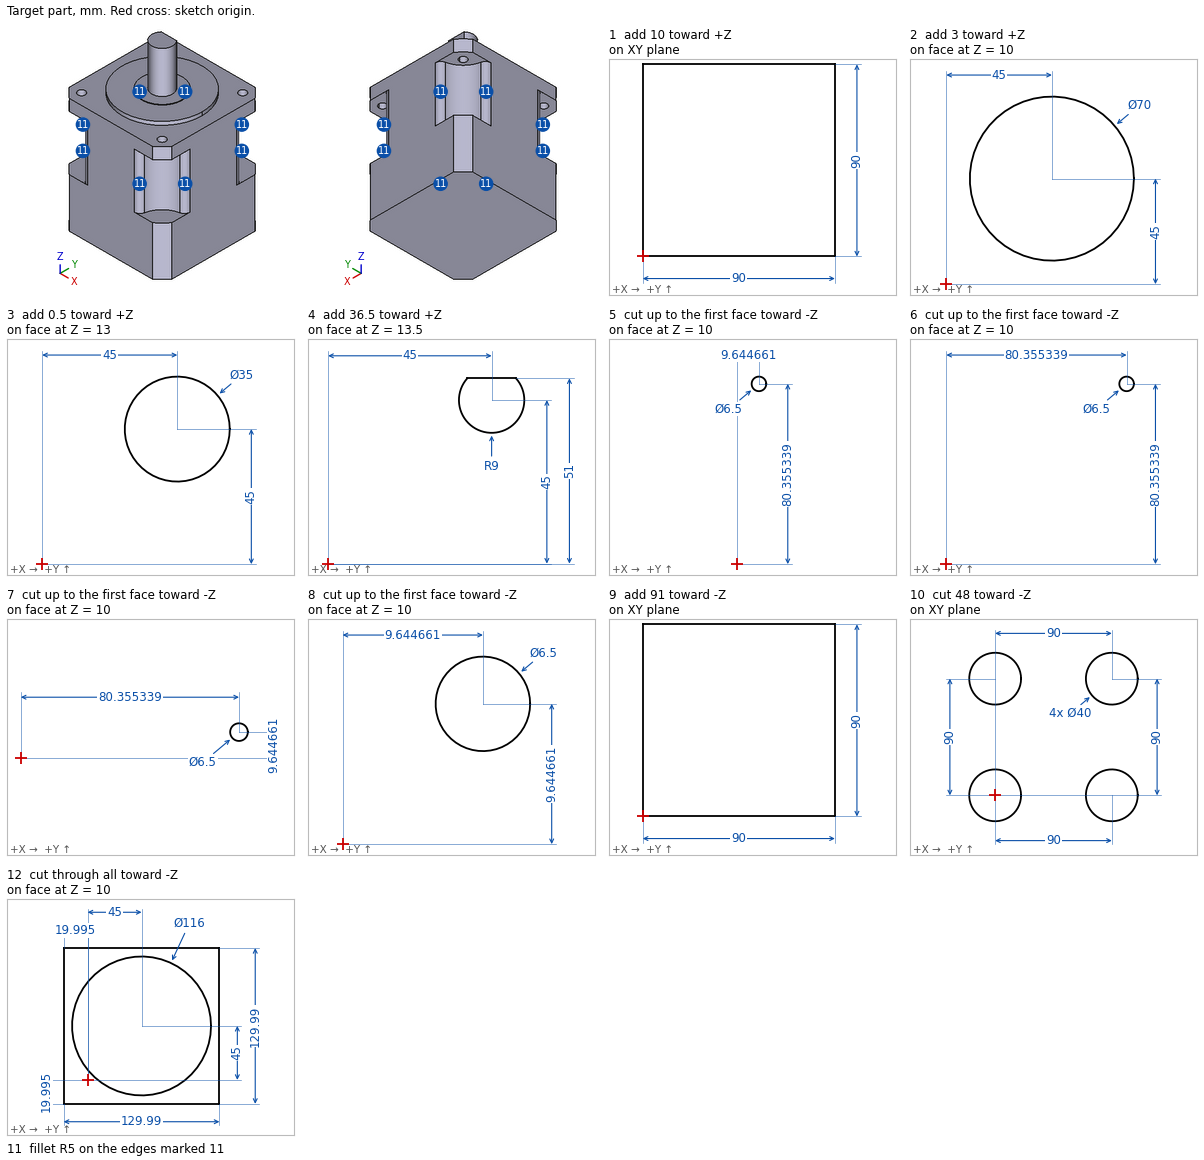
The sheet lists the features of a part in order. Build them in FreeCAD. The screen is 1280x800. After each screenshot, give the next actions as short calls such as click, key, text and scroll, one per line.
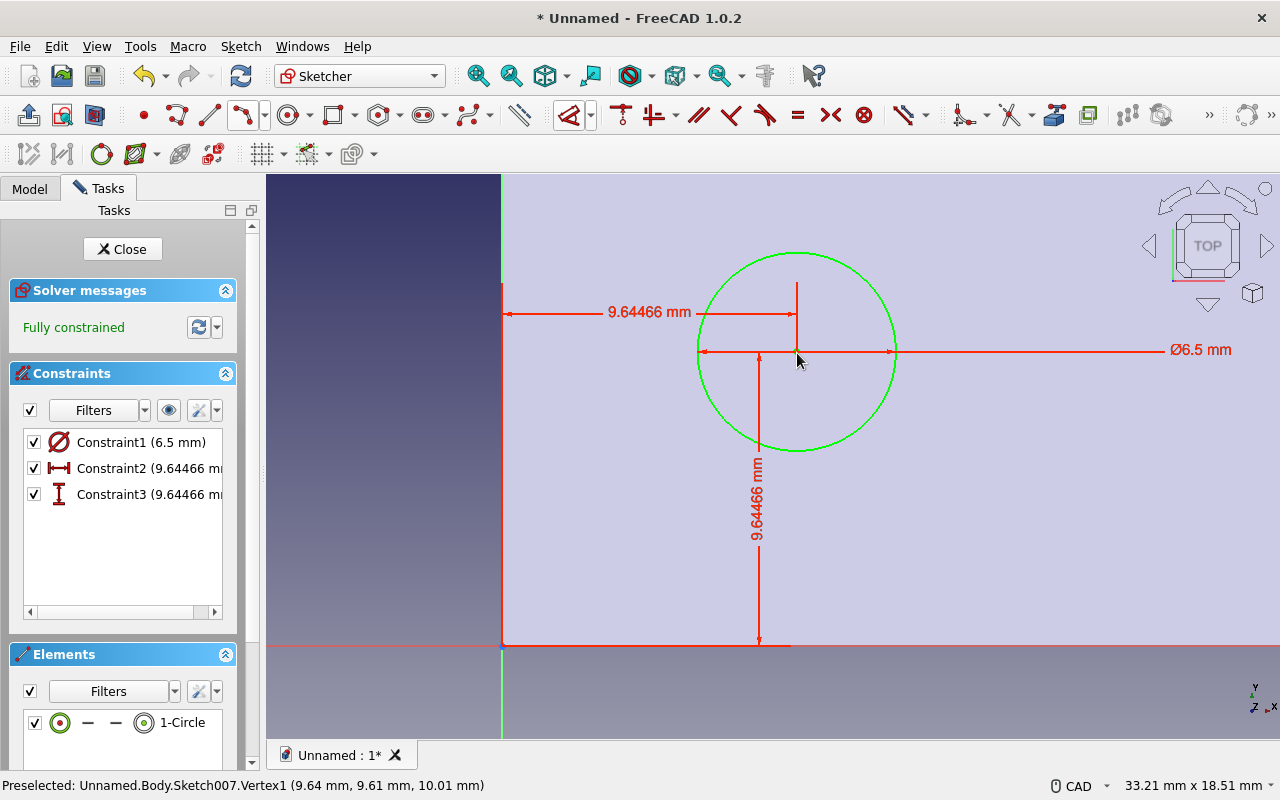
click(123, 249)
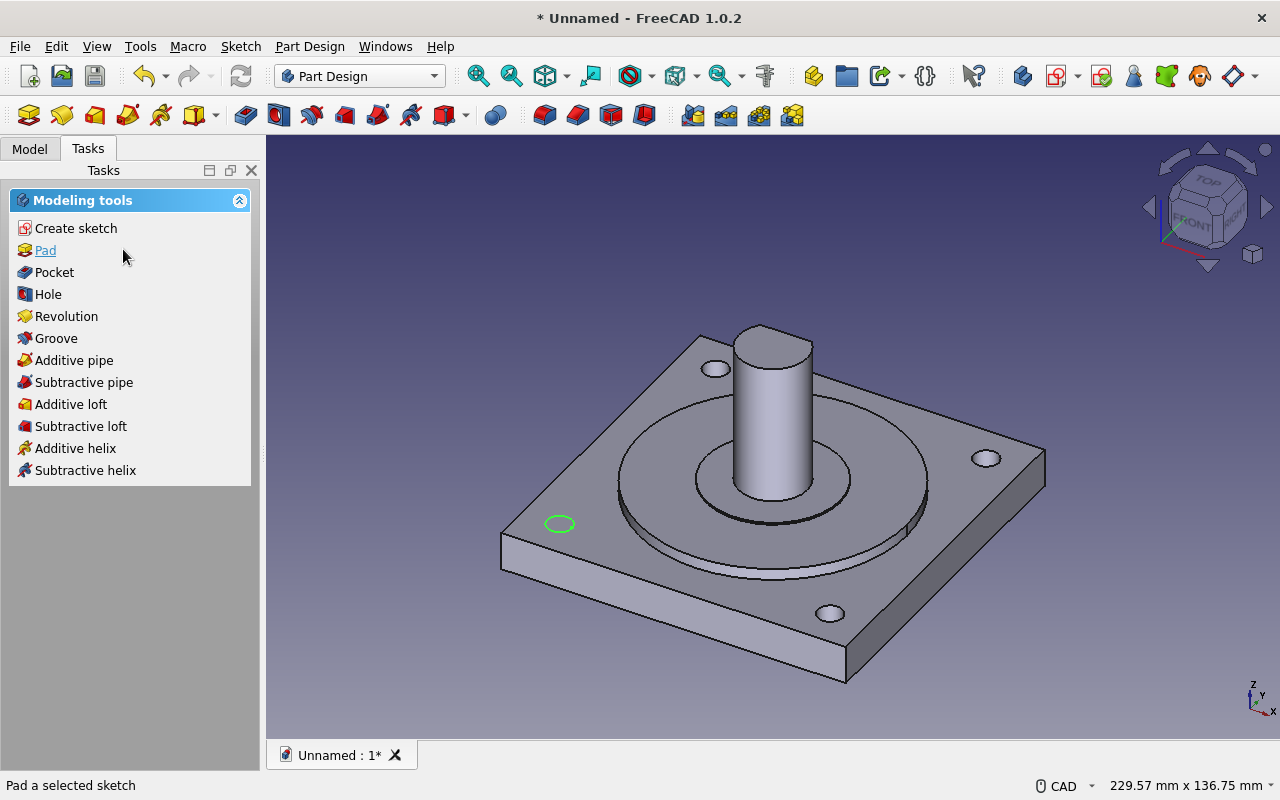
click(246, 116)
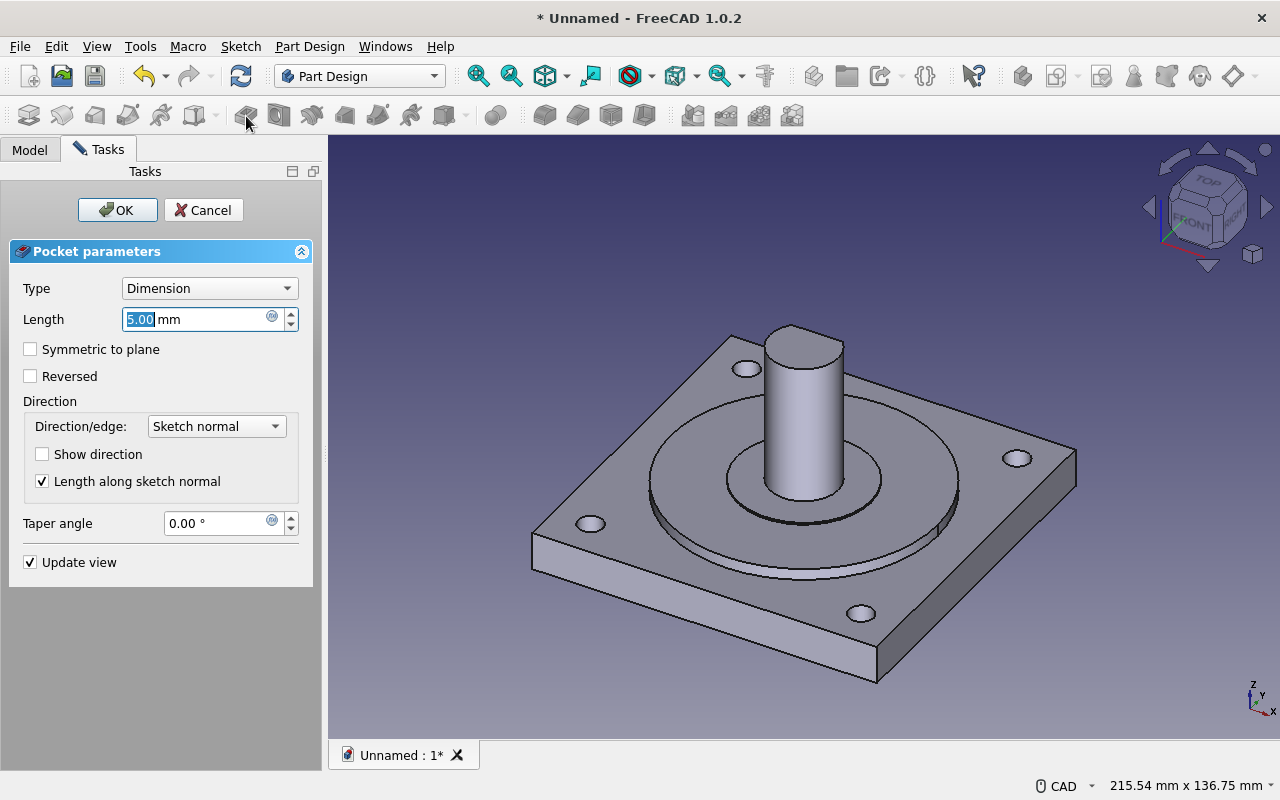
click(210, 288)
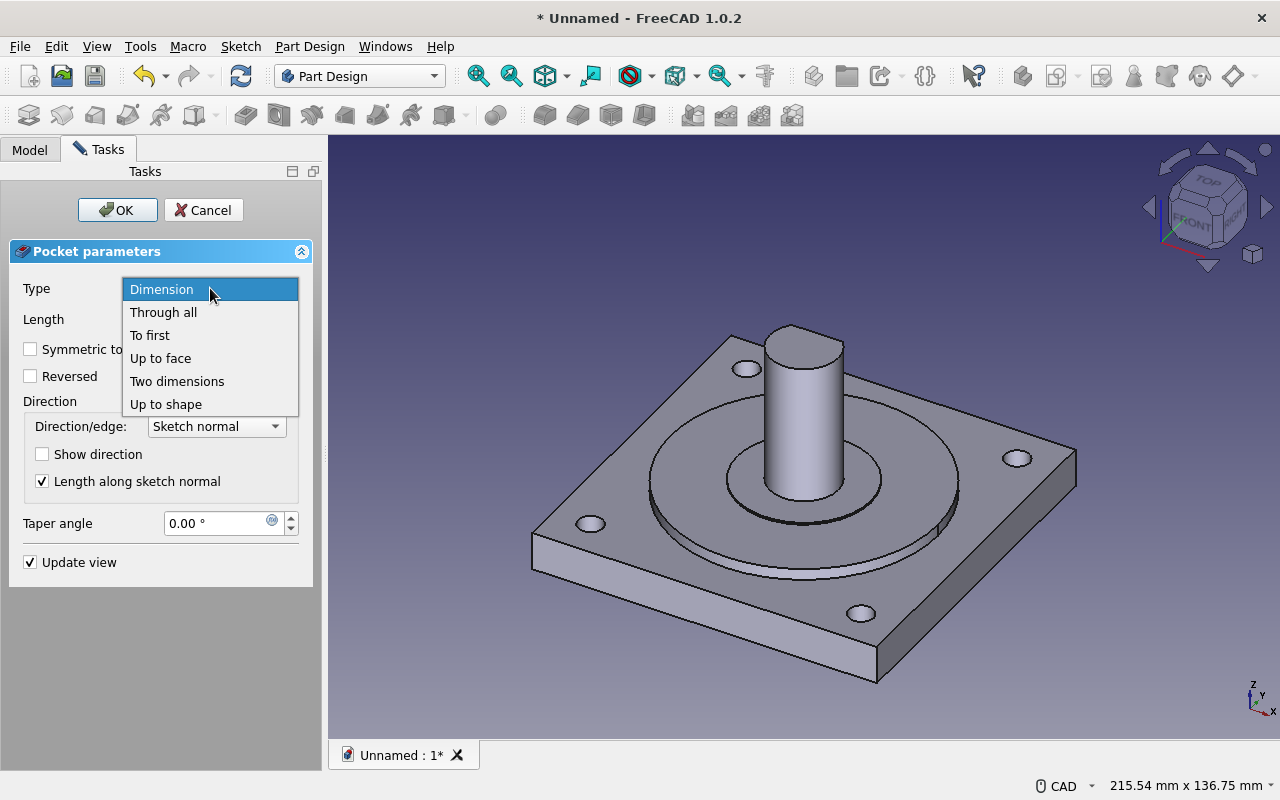
click(208, 336)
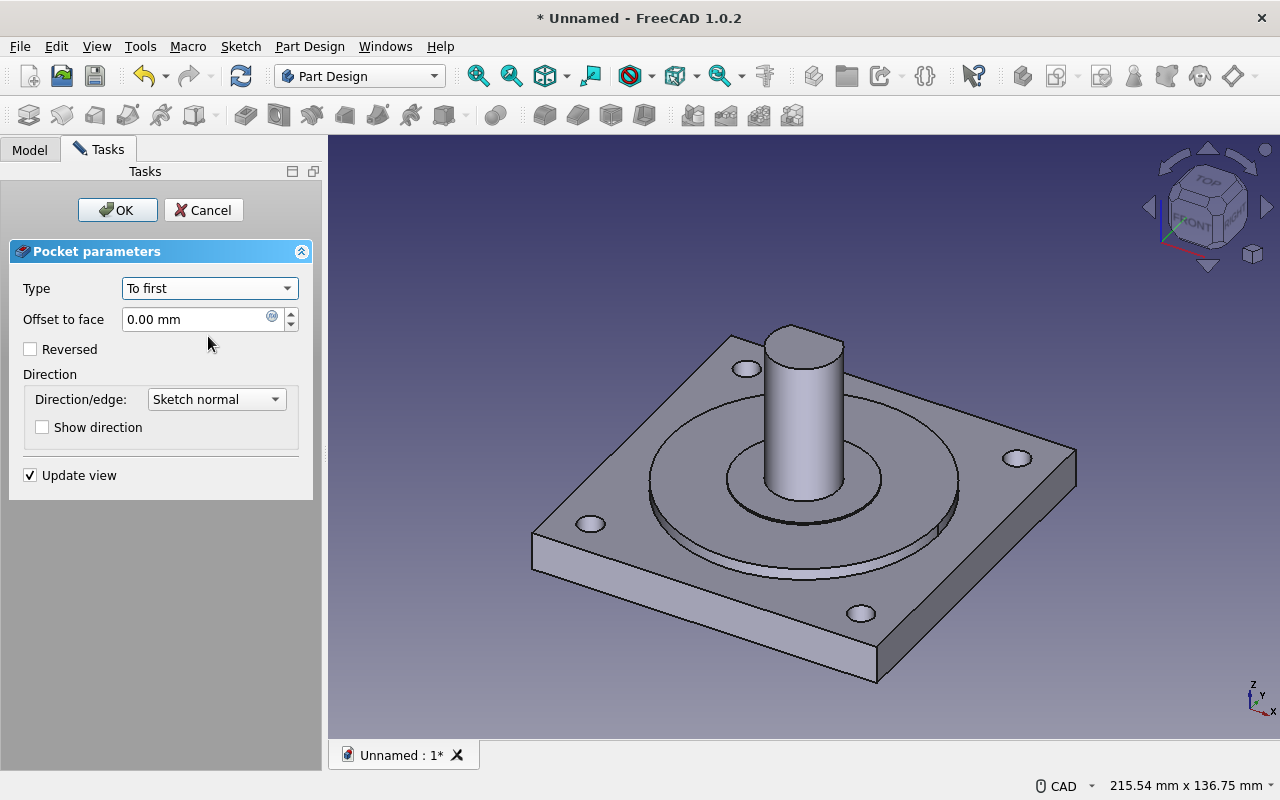
click(118, 210)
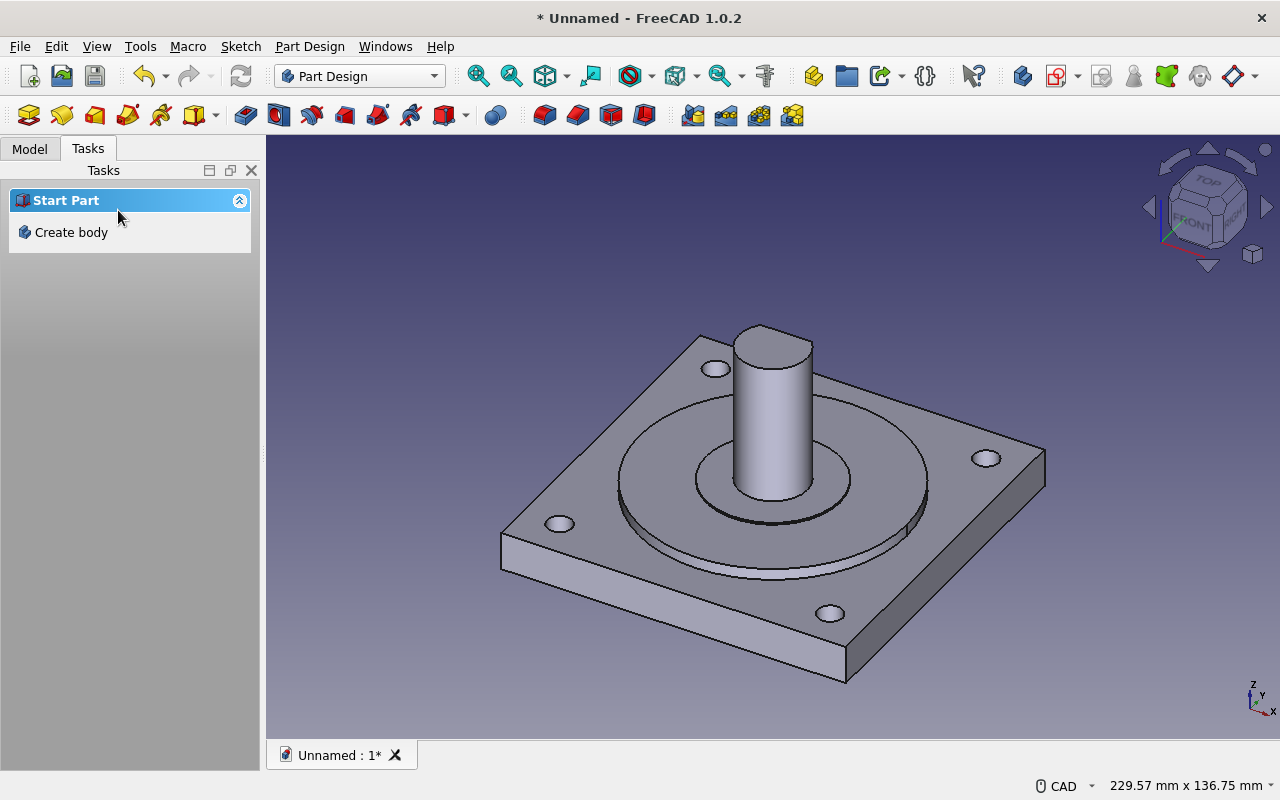
click(1056, 76)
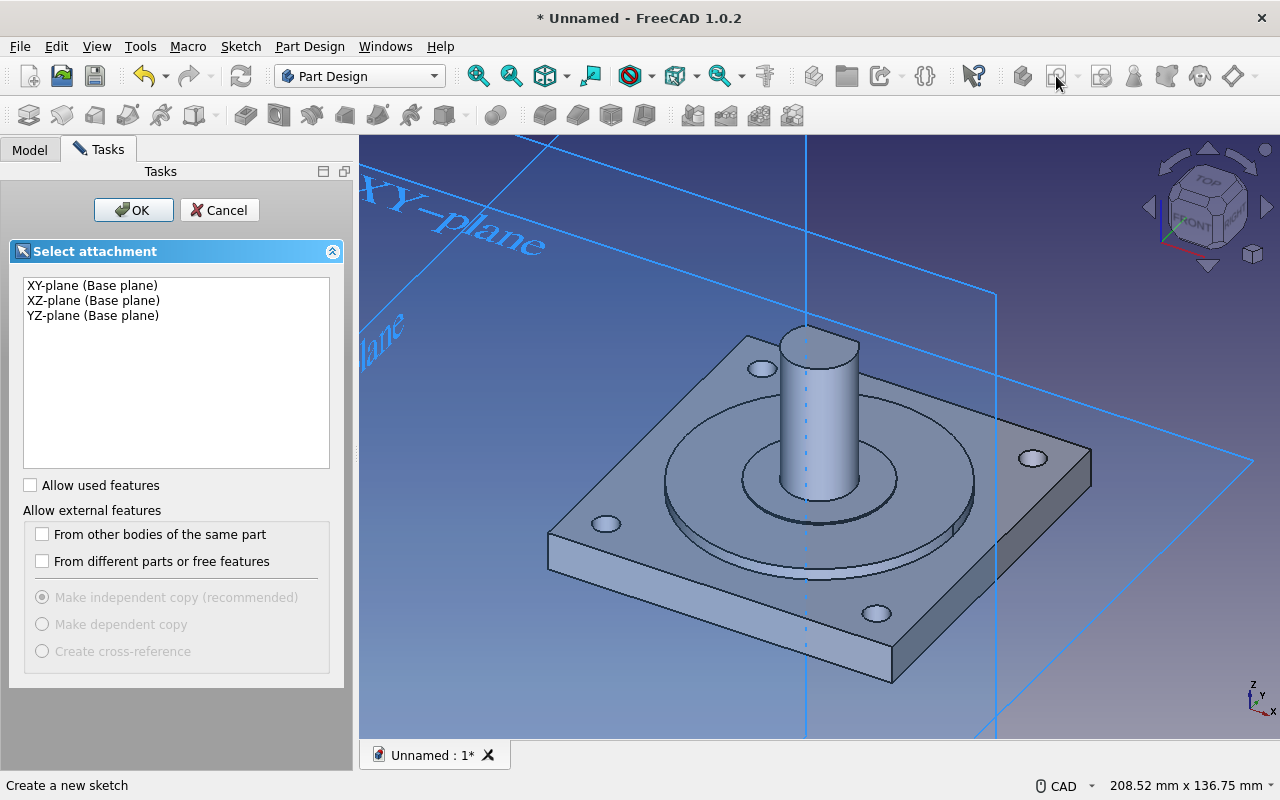
click(84, 286)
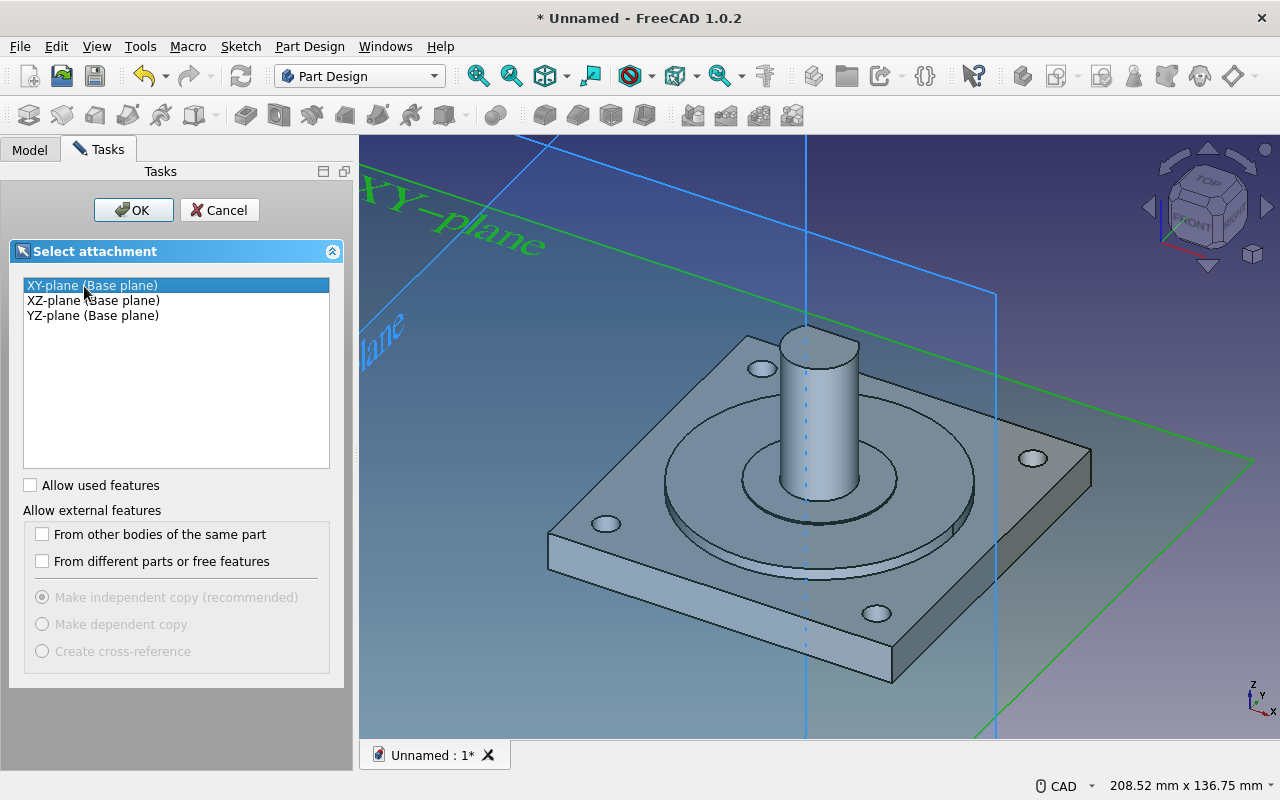
click(134, 210)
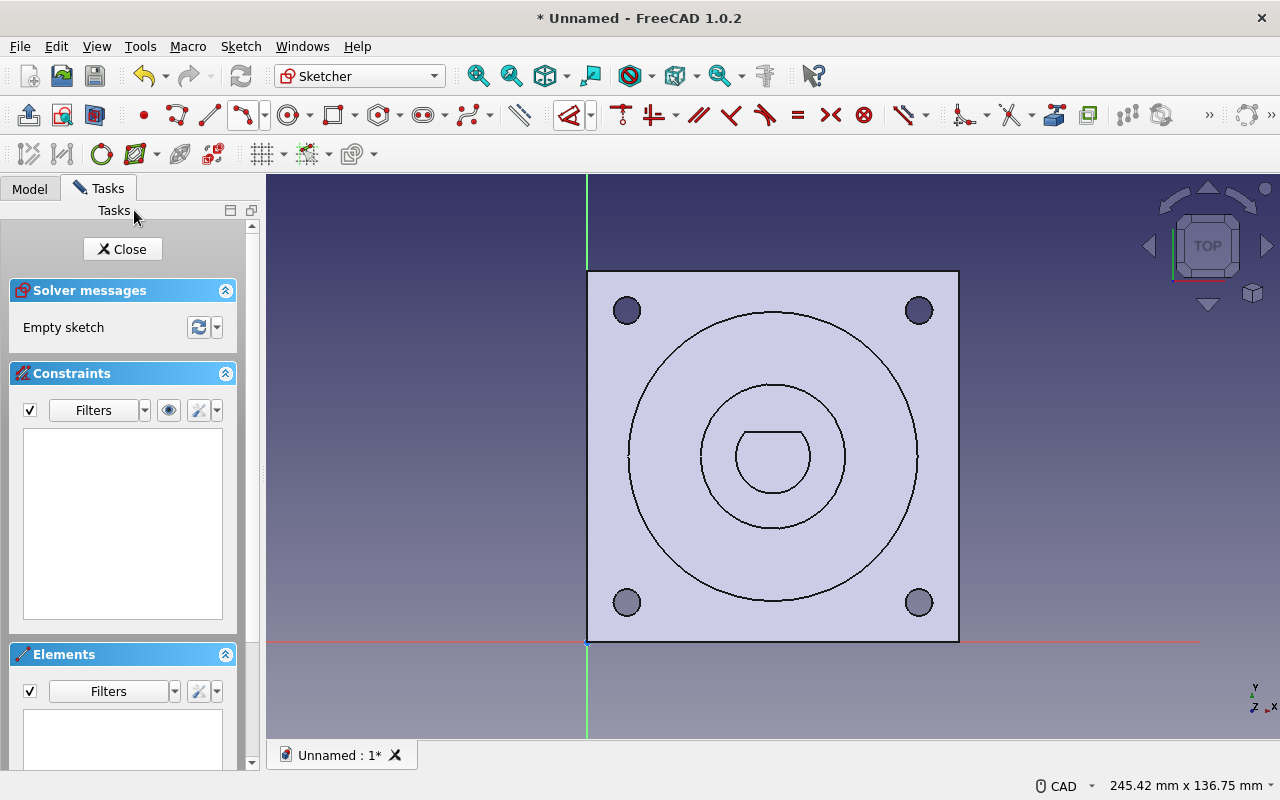
key(q)
key(s)